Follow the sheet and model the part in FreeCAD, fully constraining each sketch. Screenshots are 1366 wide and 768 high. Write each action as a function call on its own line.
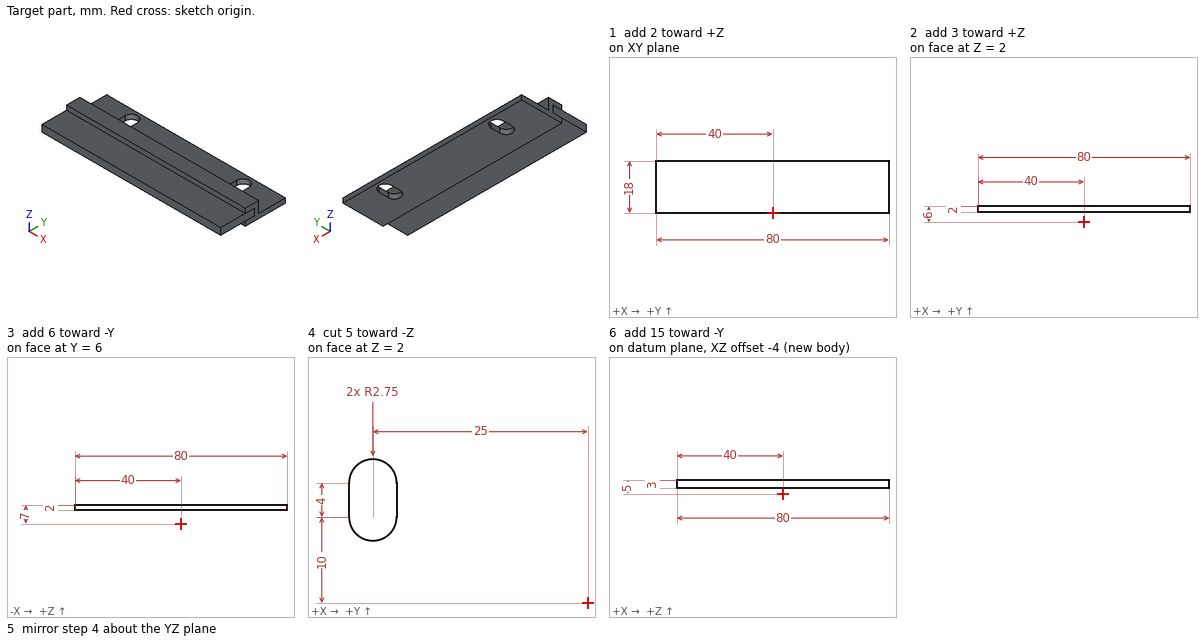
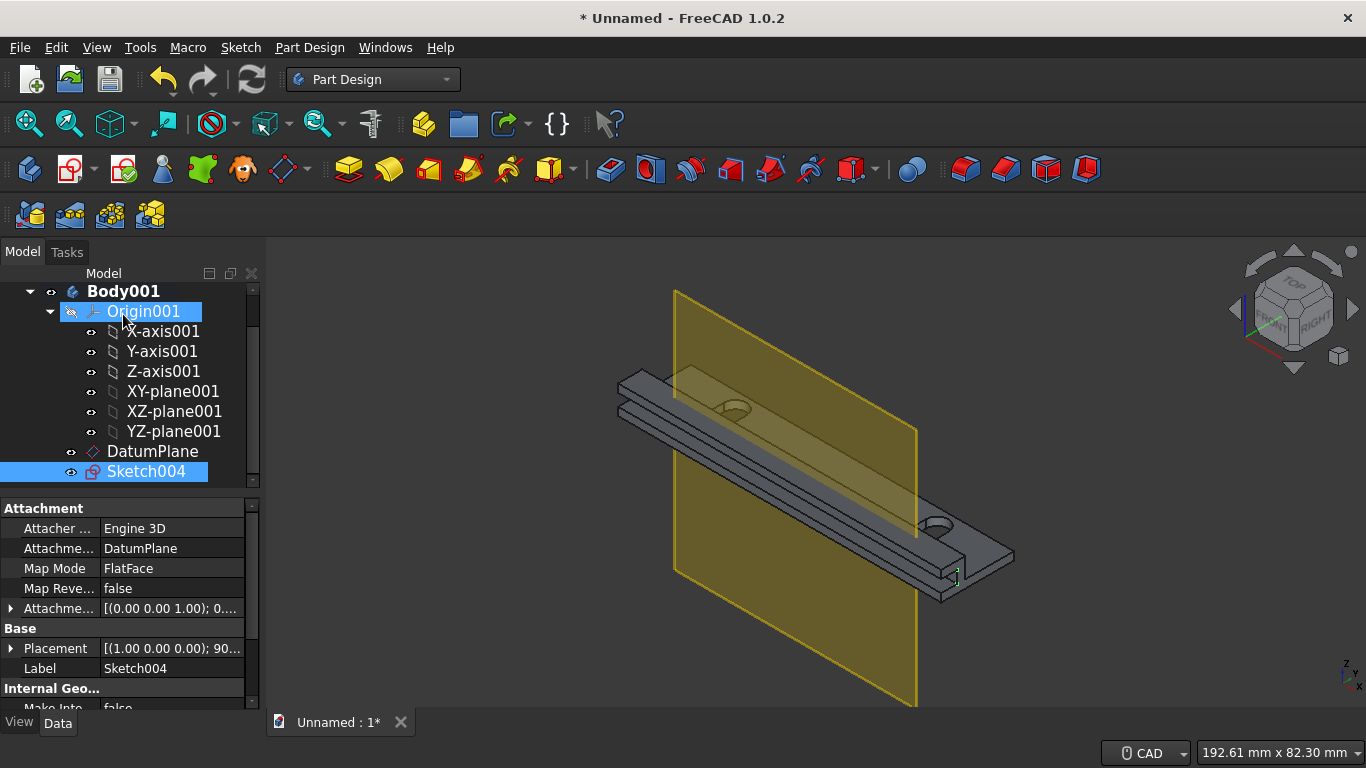
click(350, 170)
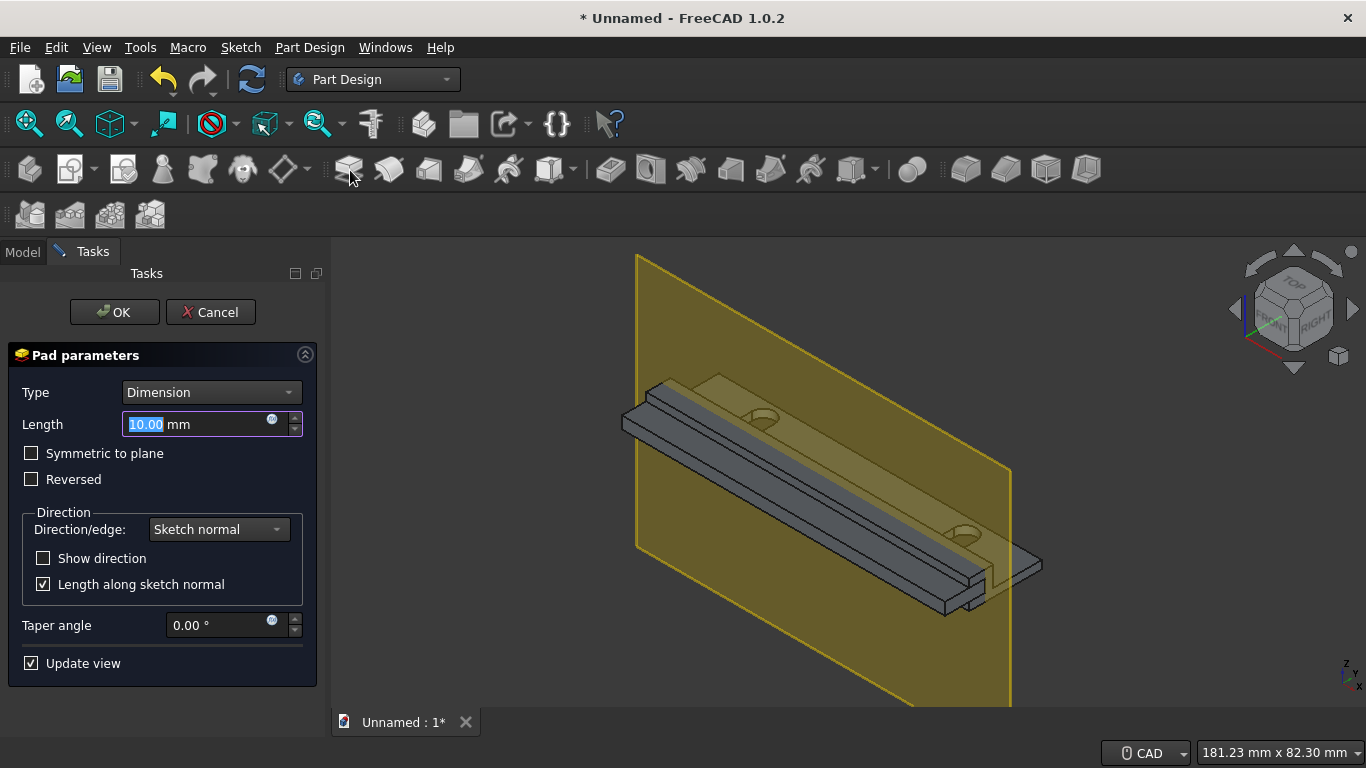
text(15)
key(Tab)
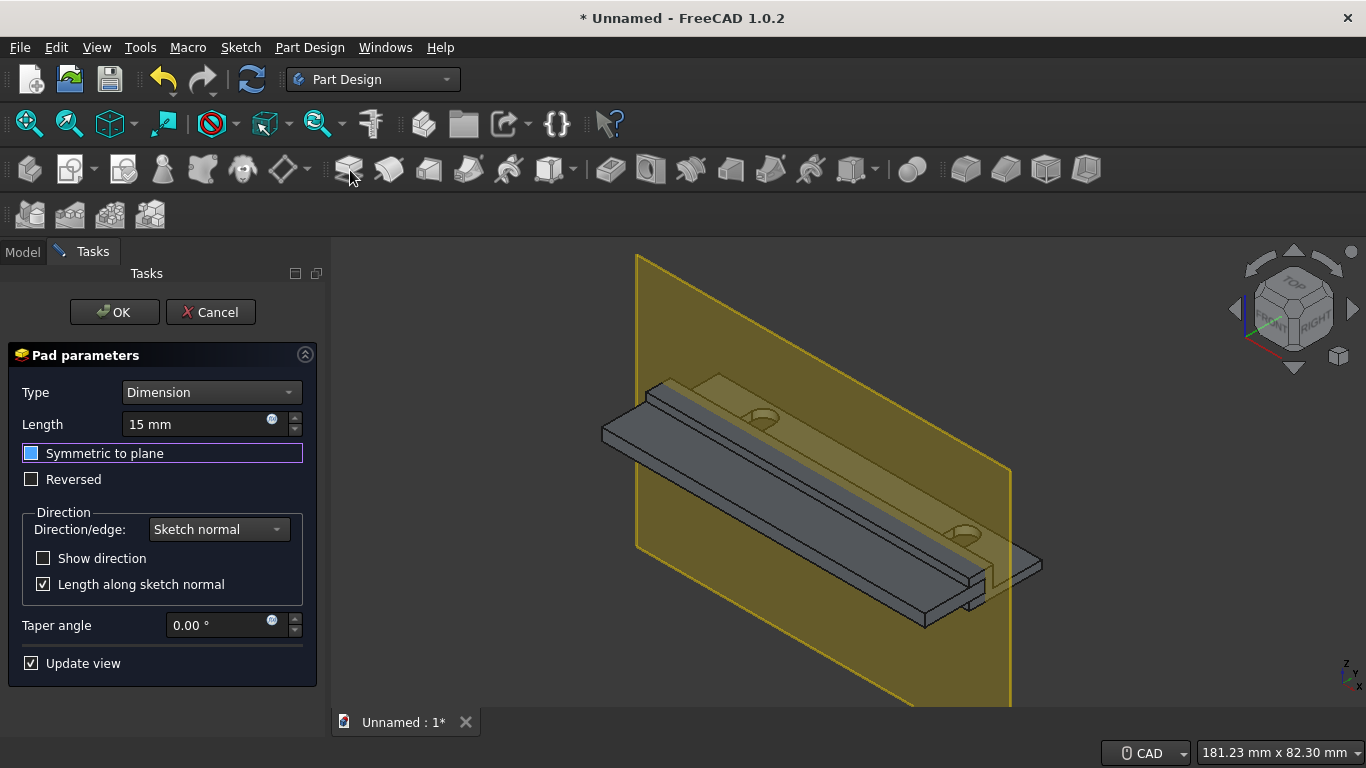
click(115, 312)